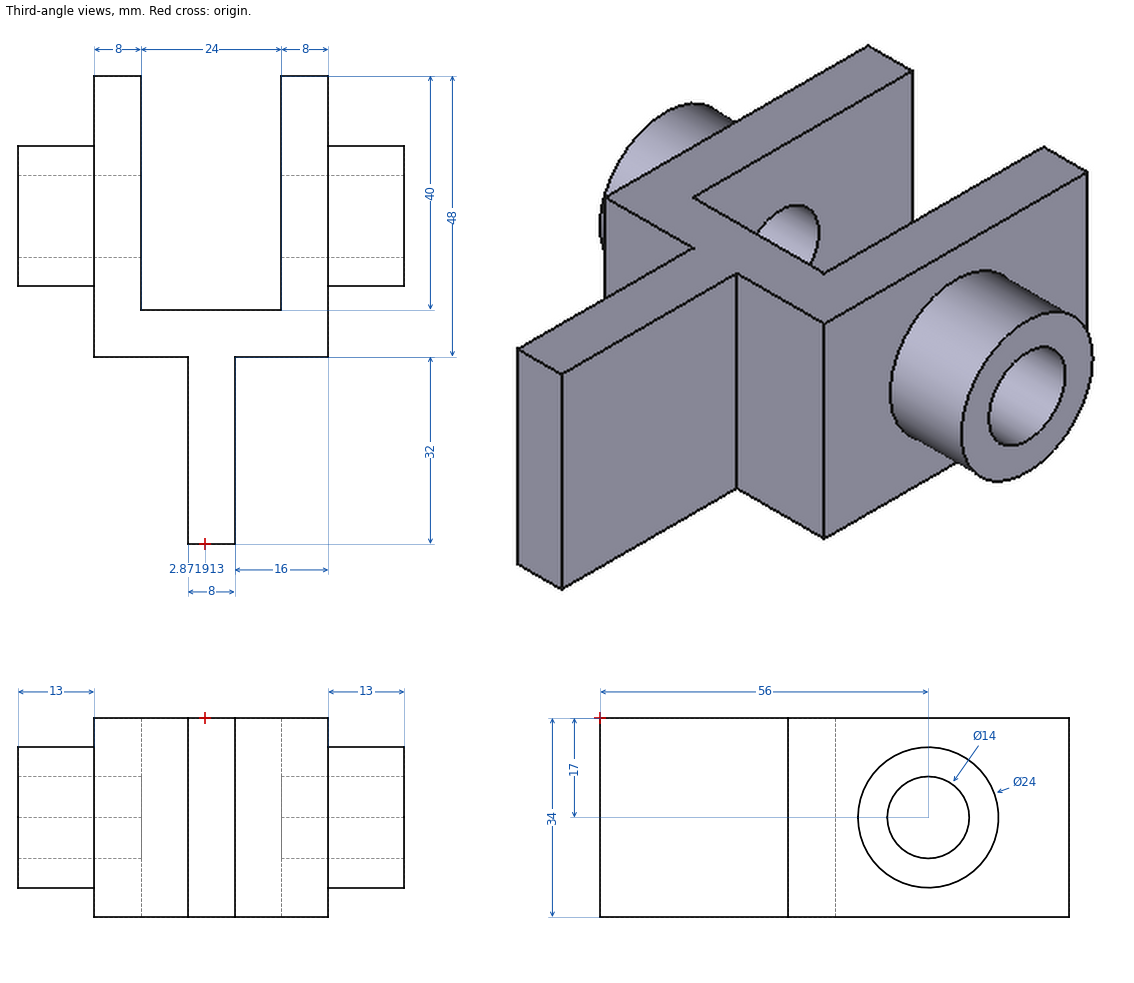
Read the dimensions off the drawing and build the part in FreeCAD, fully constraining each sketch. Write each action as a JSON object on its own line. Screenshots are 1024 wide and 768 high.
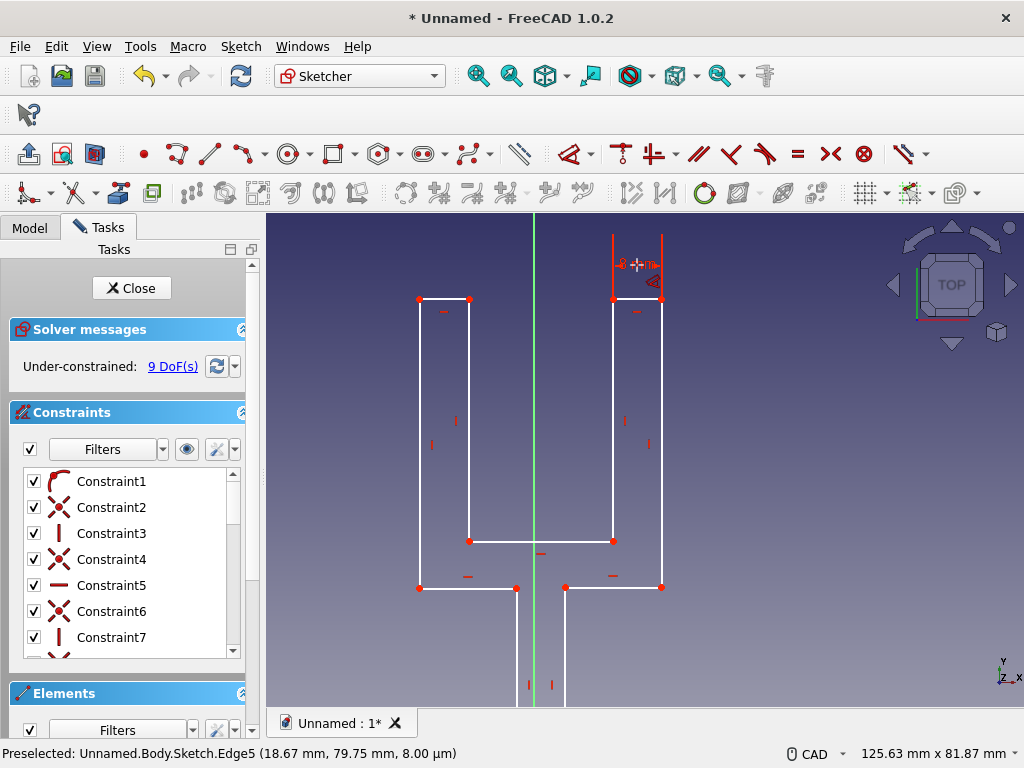
{"action": "left_click", "coordinate": [454, 299]}
{"action": "left_click", "coordinate": [444, 265]}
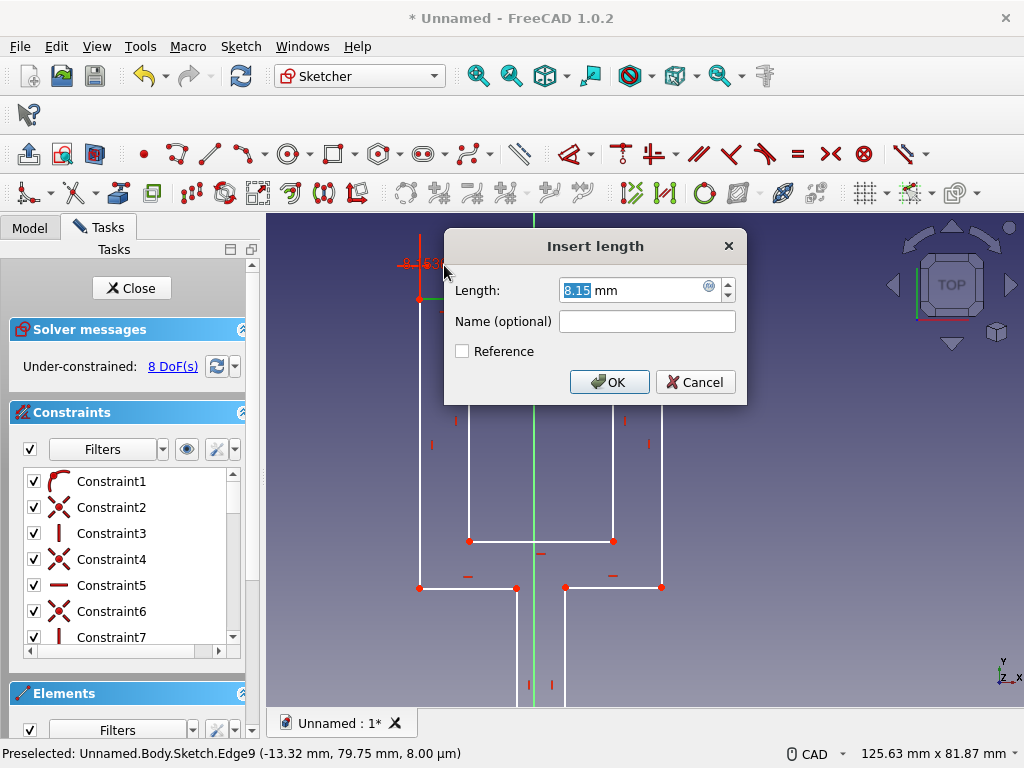
{"action": "type", "text": "8"}
{"action": "key", "text": "Return"}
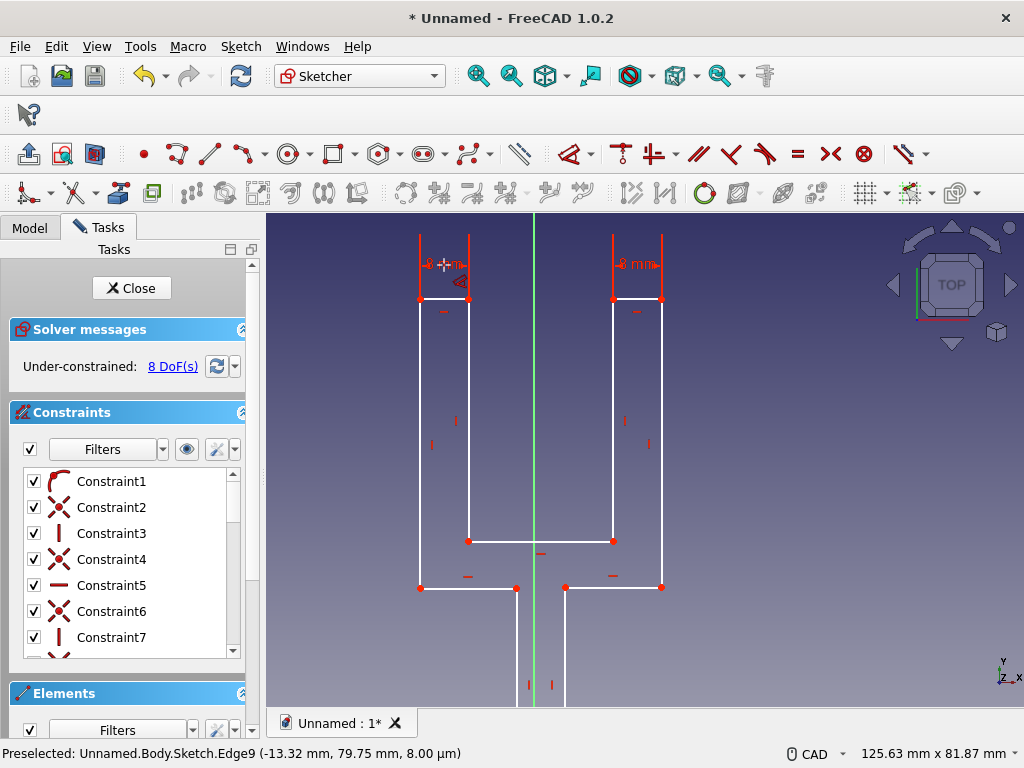
{"action": "left_click", "coordinate": [565, 646]}
{"action": "left_click", "coordinate": [599, 633]}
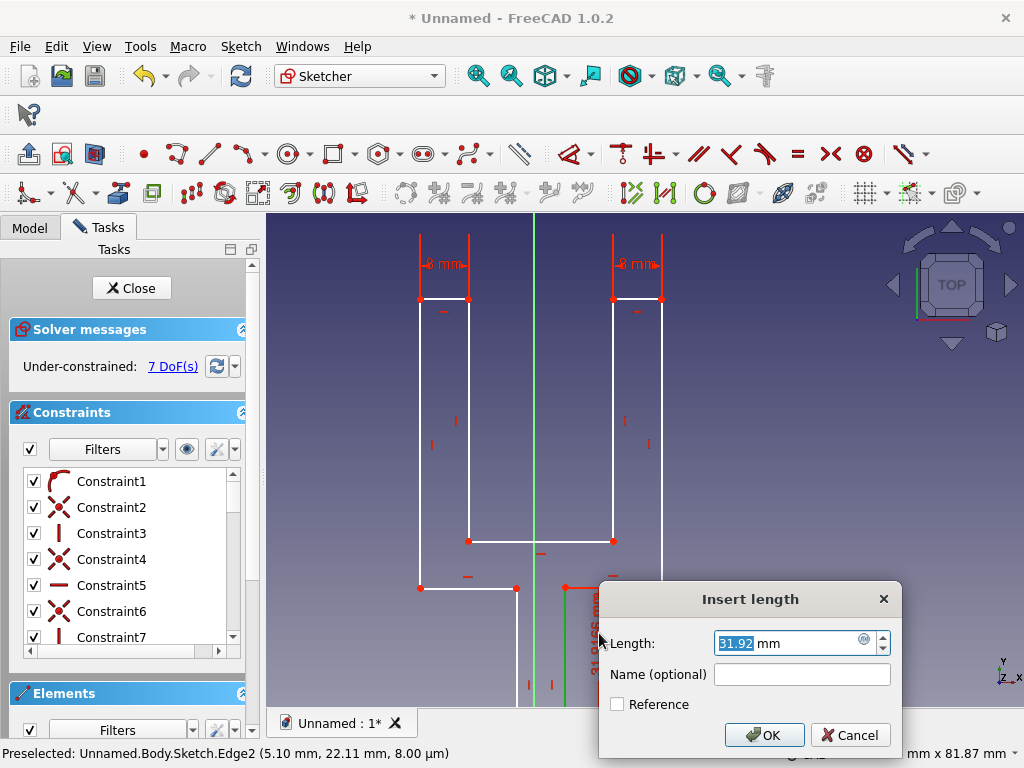
{"action": "type", "text": "32"}
{"action": "key", "text": "Return"}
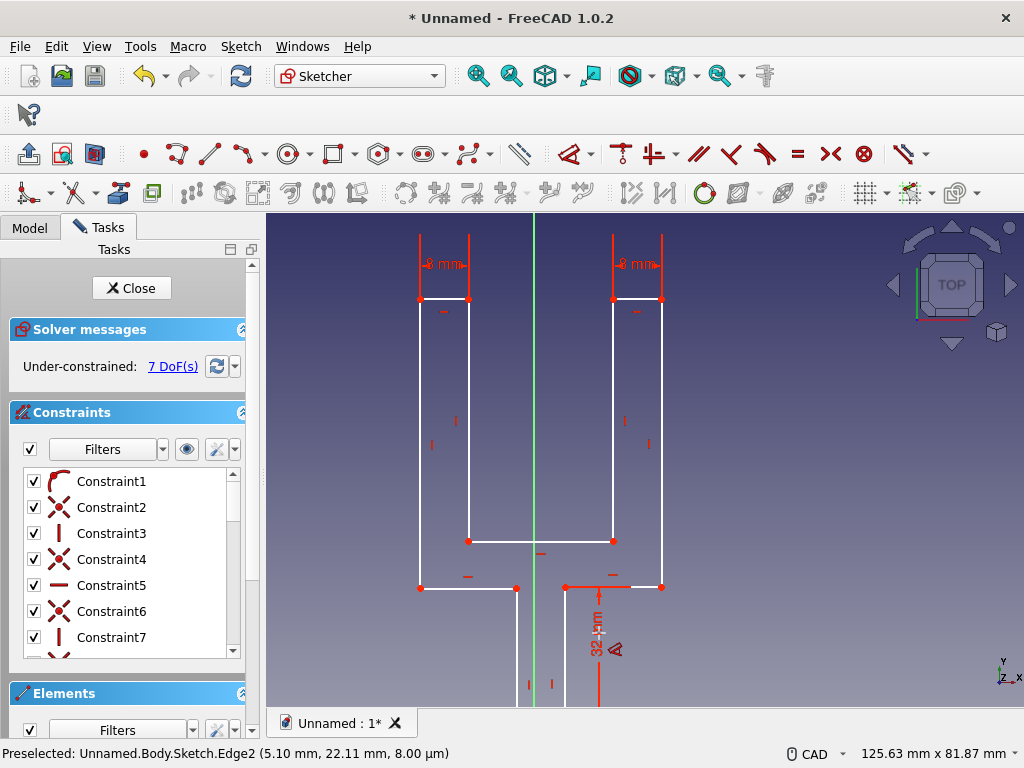
{"action": "left_click", "coordinate": [594, 587]}
{"action": "left_click", "coordinate": [636, 553]}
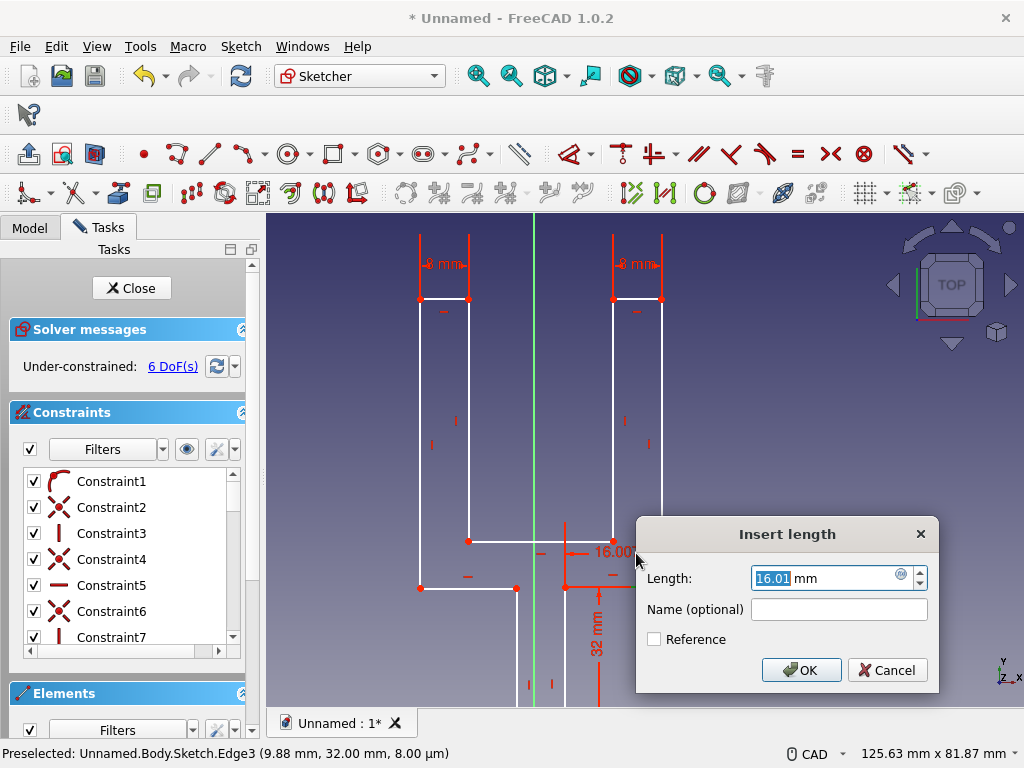
{"action": "type", "text": "16"}
{"action": "key", "text": "Return"}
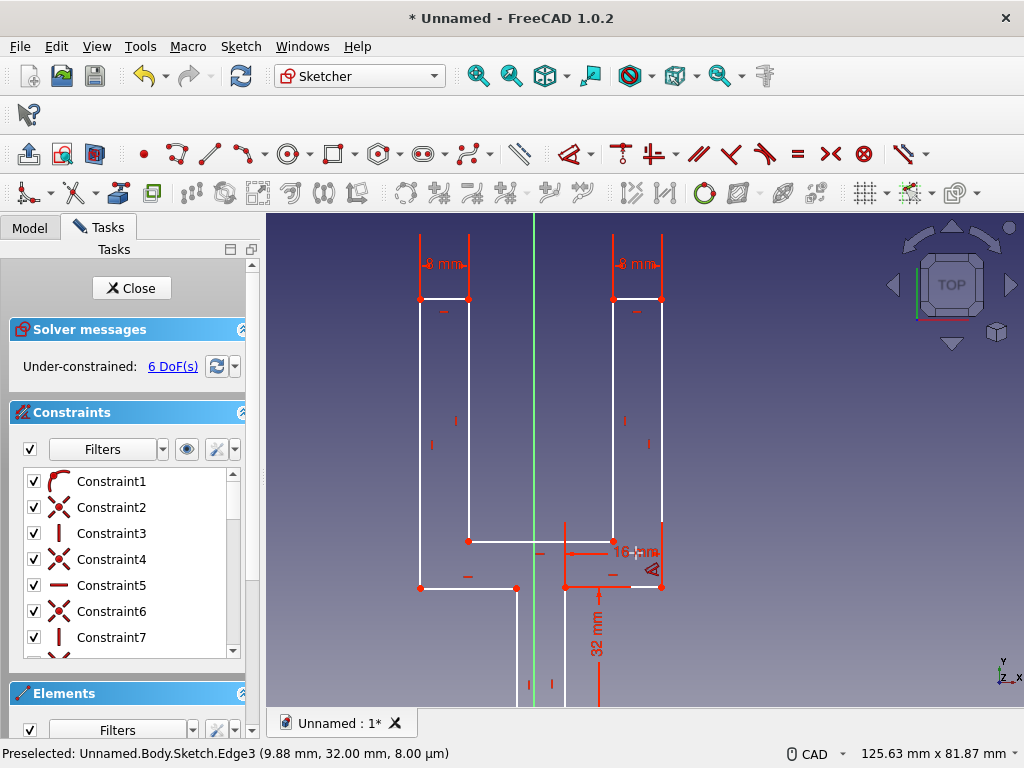
{"action": "left_click", "coordinate": [662, 501]}
{"action": "left_click", "coordinate": [696, 443]}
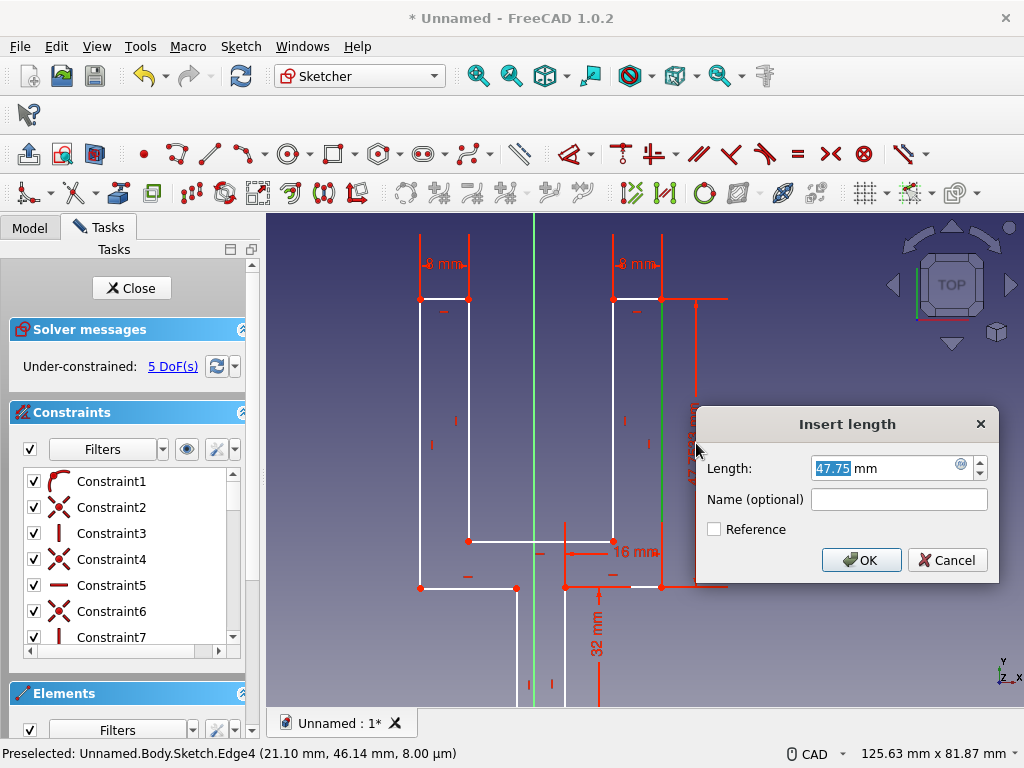
{"action": "type", "text": "48"}
{"action": "key", "text": "Return"}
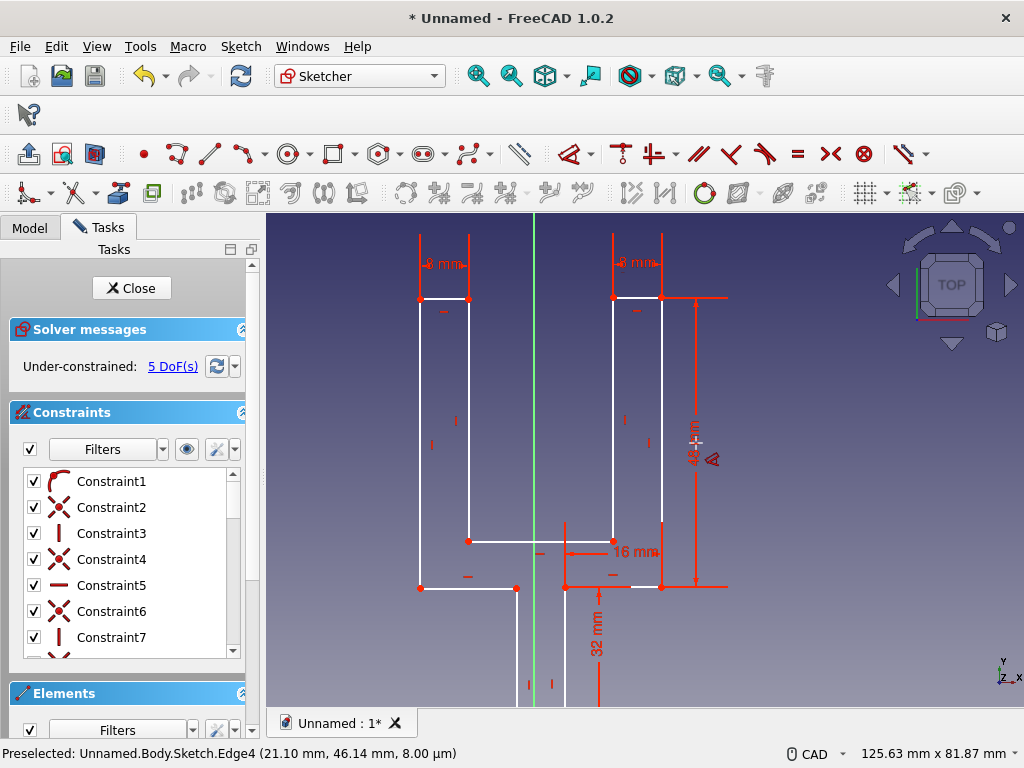
{"action": "left_click", "coordinate": [613, 371]}
{"action": "left_click", "coordinate": [647, 420]}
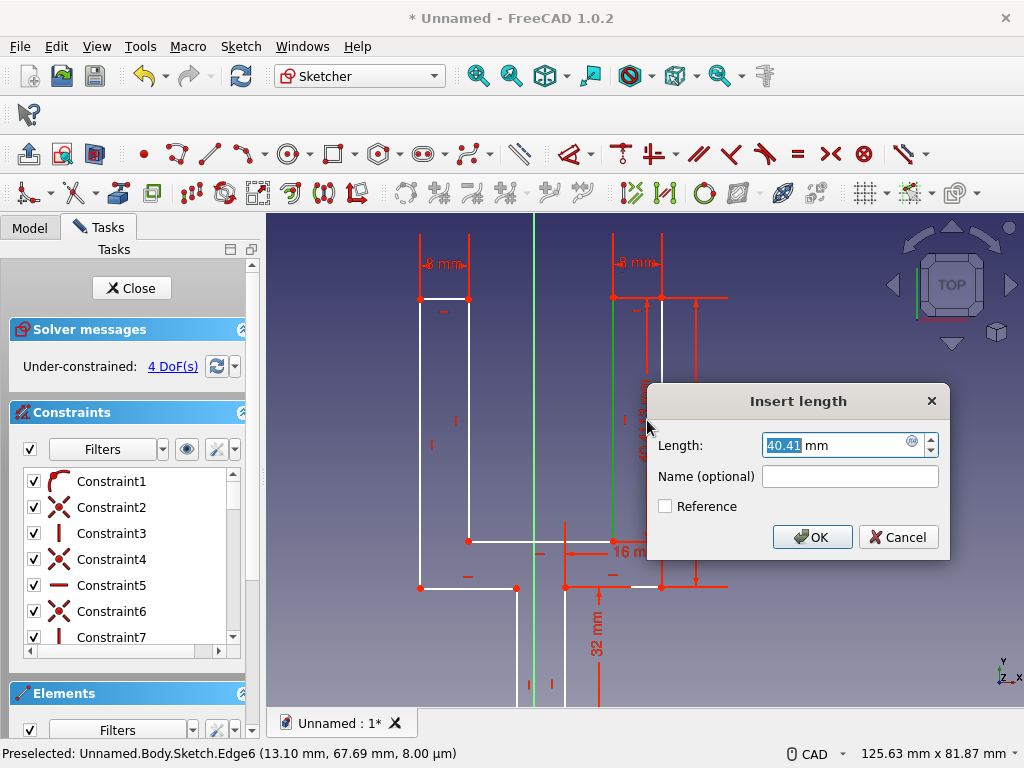
{"action": "type", "text": "40"}
{"action": "key", "text": "Return"}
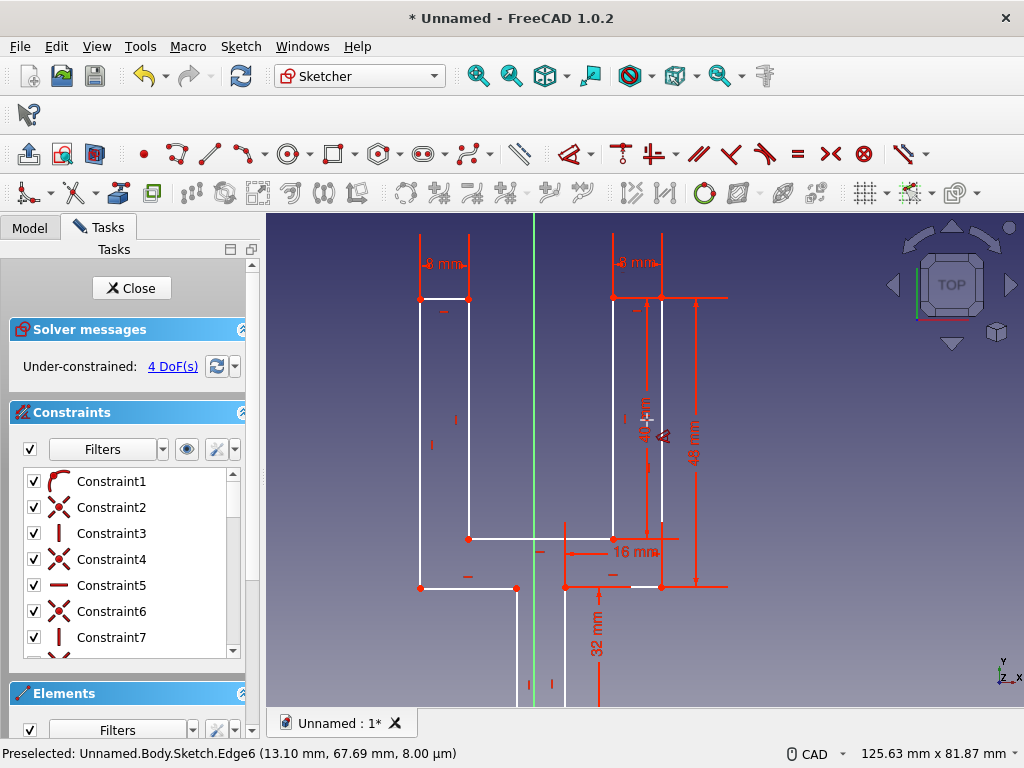
{"action": "left_click", "coordinate": [570, 539]}
{"action": "left_click", "coordinate": [508, 573]}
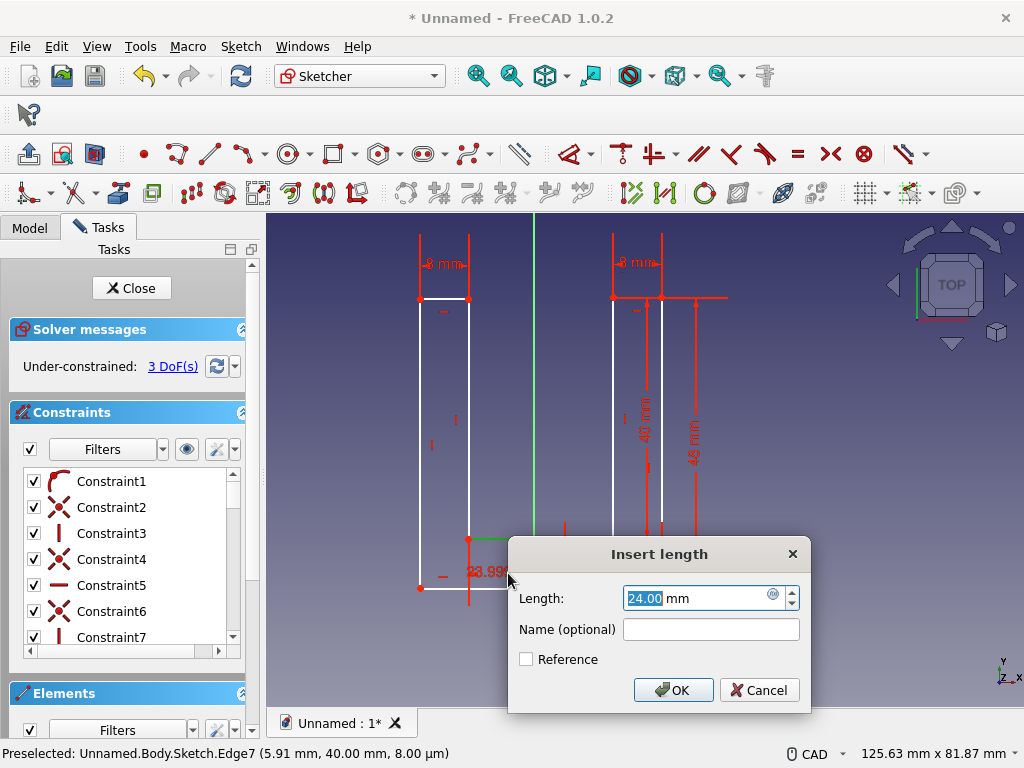
{"action": "type", "text": "24"}
{"action": "key", "text": "Return"}